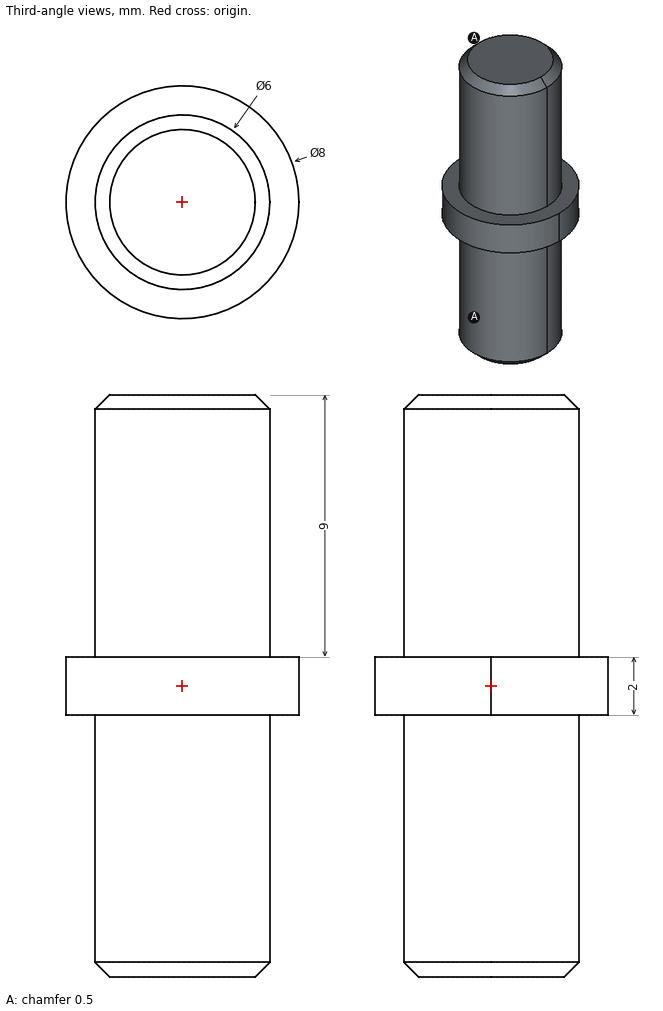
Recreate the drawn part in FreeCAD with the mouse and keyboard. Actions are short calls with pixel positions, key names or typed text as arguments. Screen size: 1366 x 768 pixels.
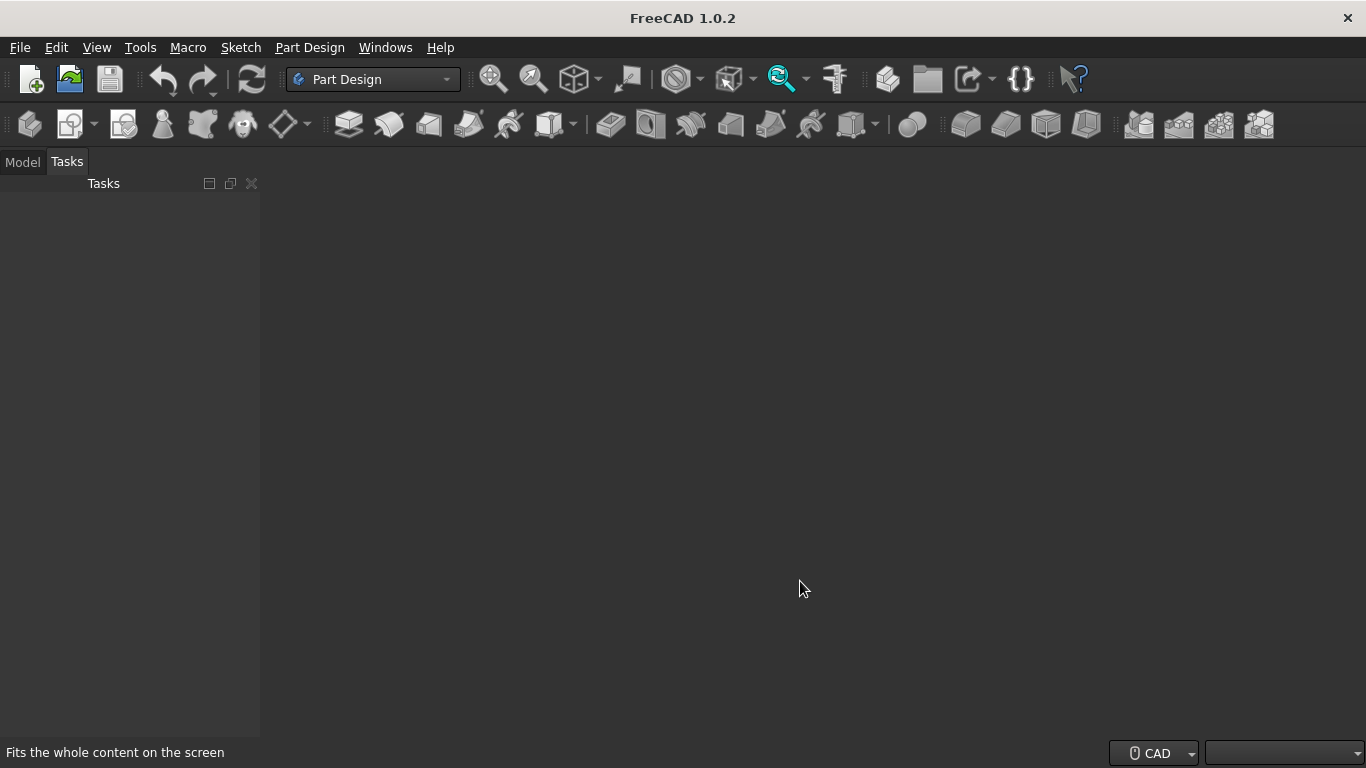
click(30, 80)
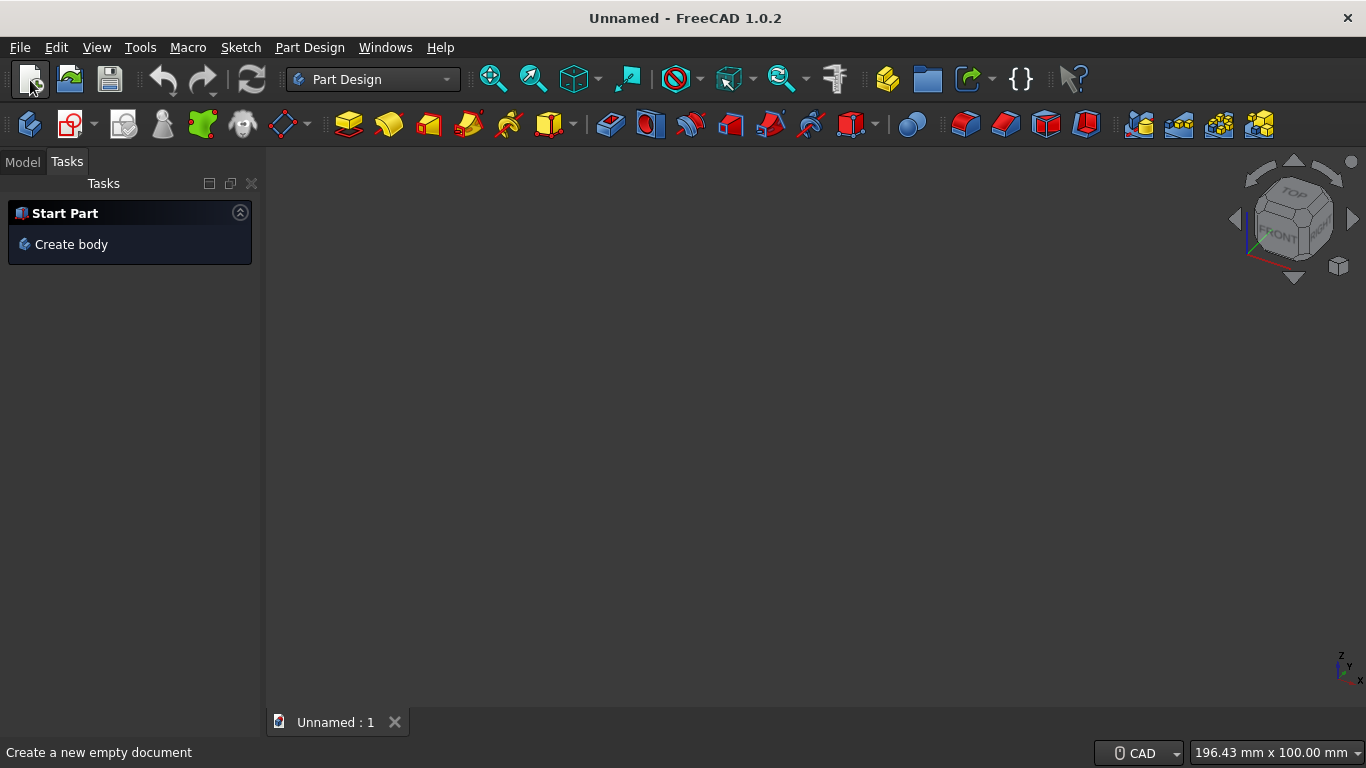
click(70, 124)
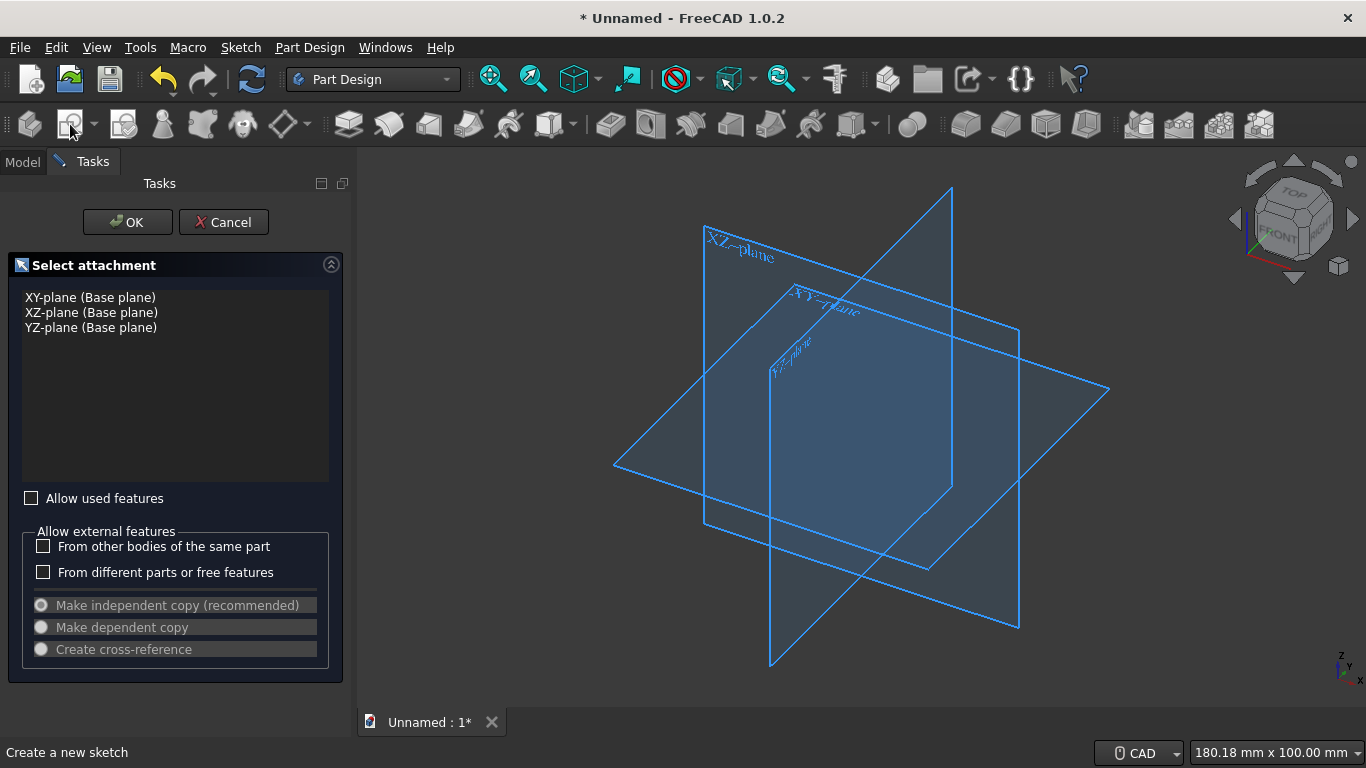
click(82, 298)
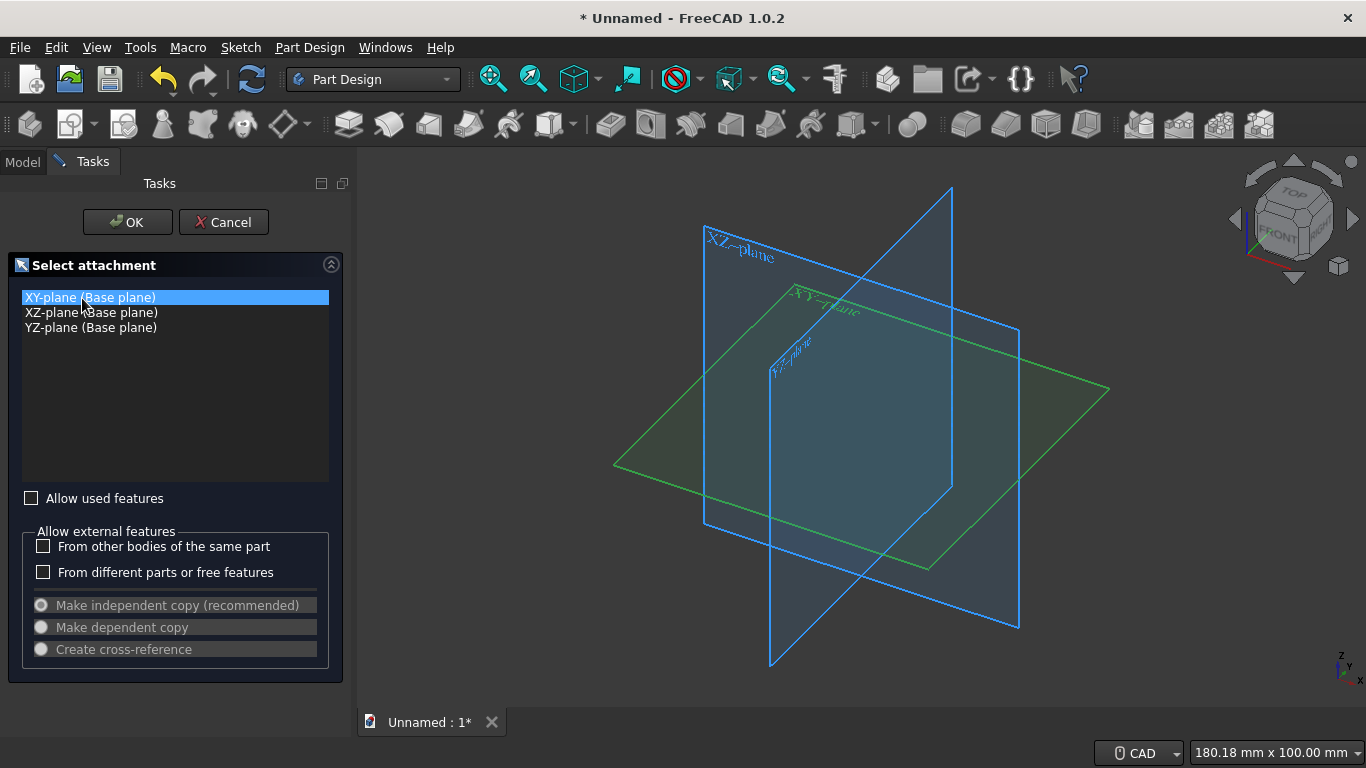
click(128, 222)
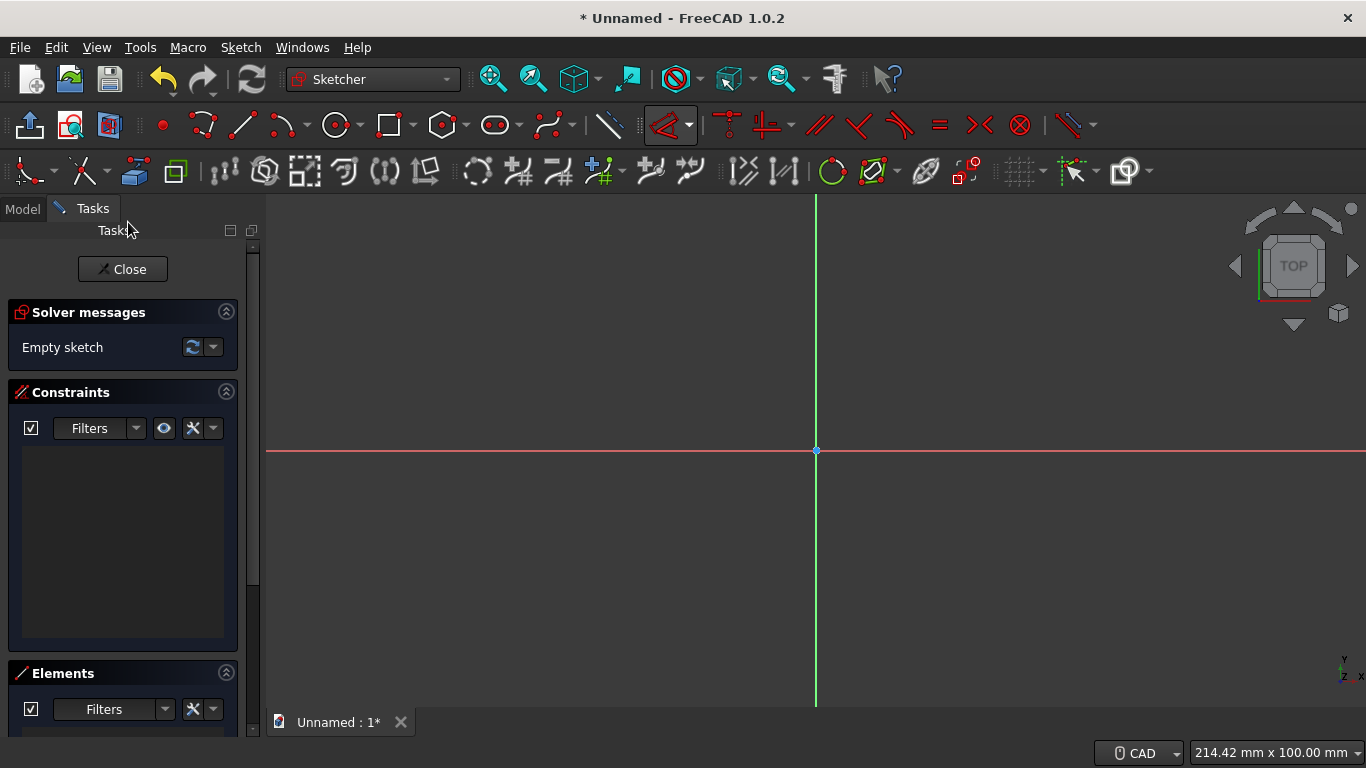
scroll(827, 450, up, 10)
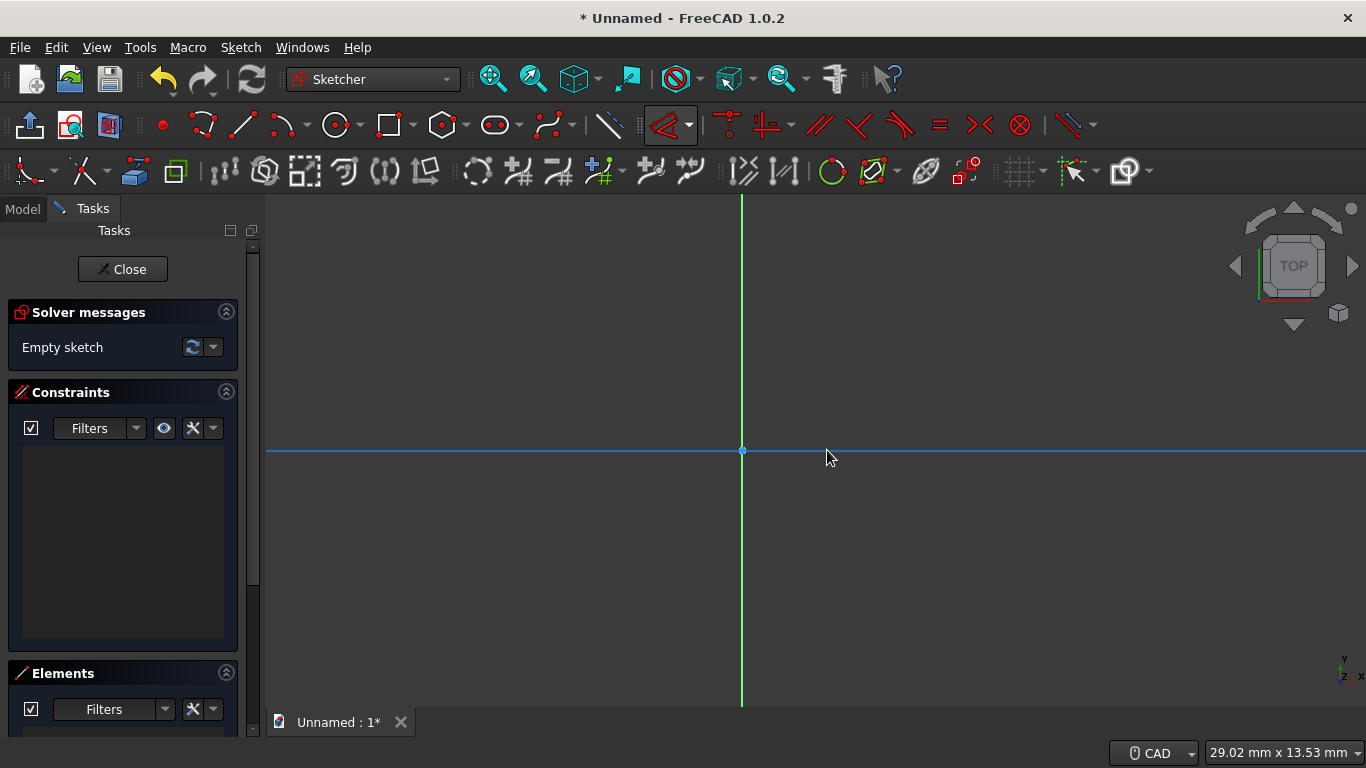
key(g)
key(c)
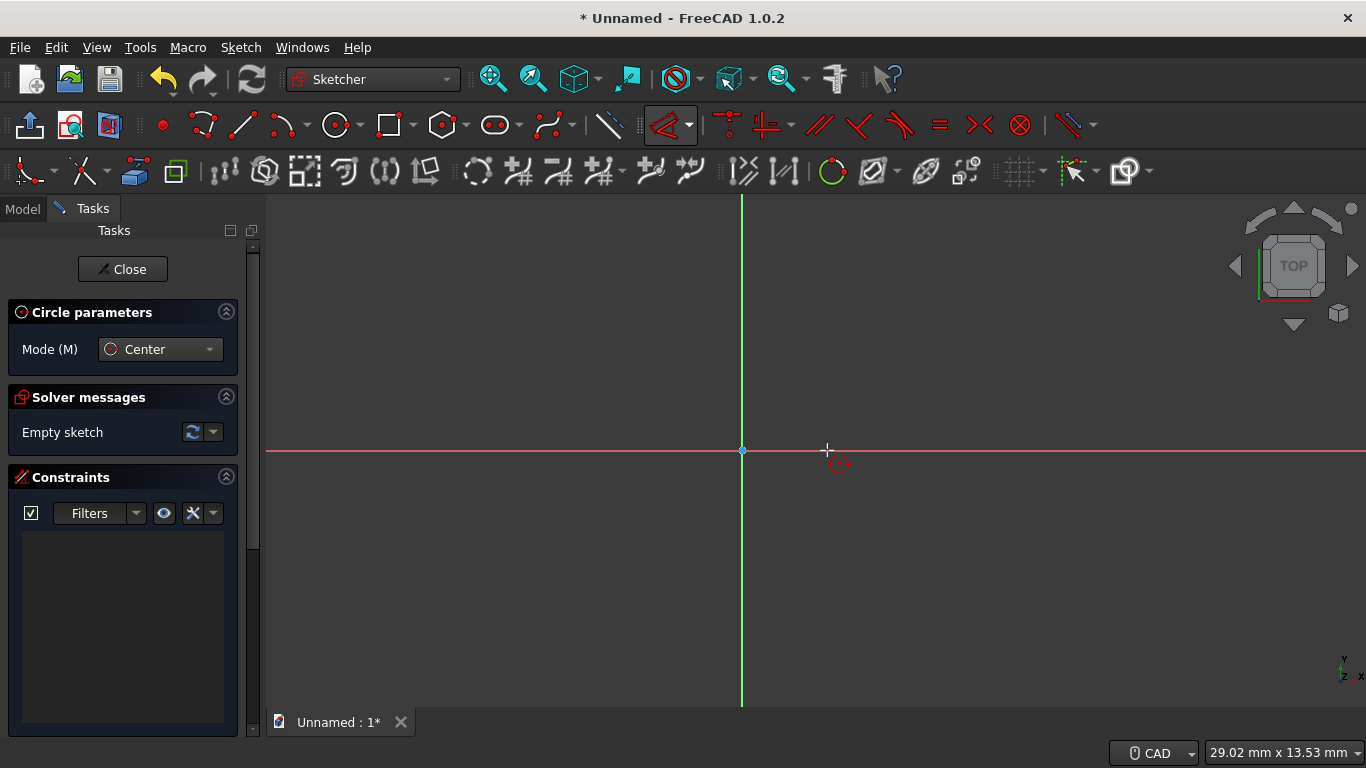
click(742, 450)
click(850, 343)
key(Escape)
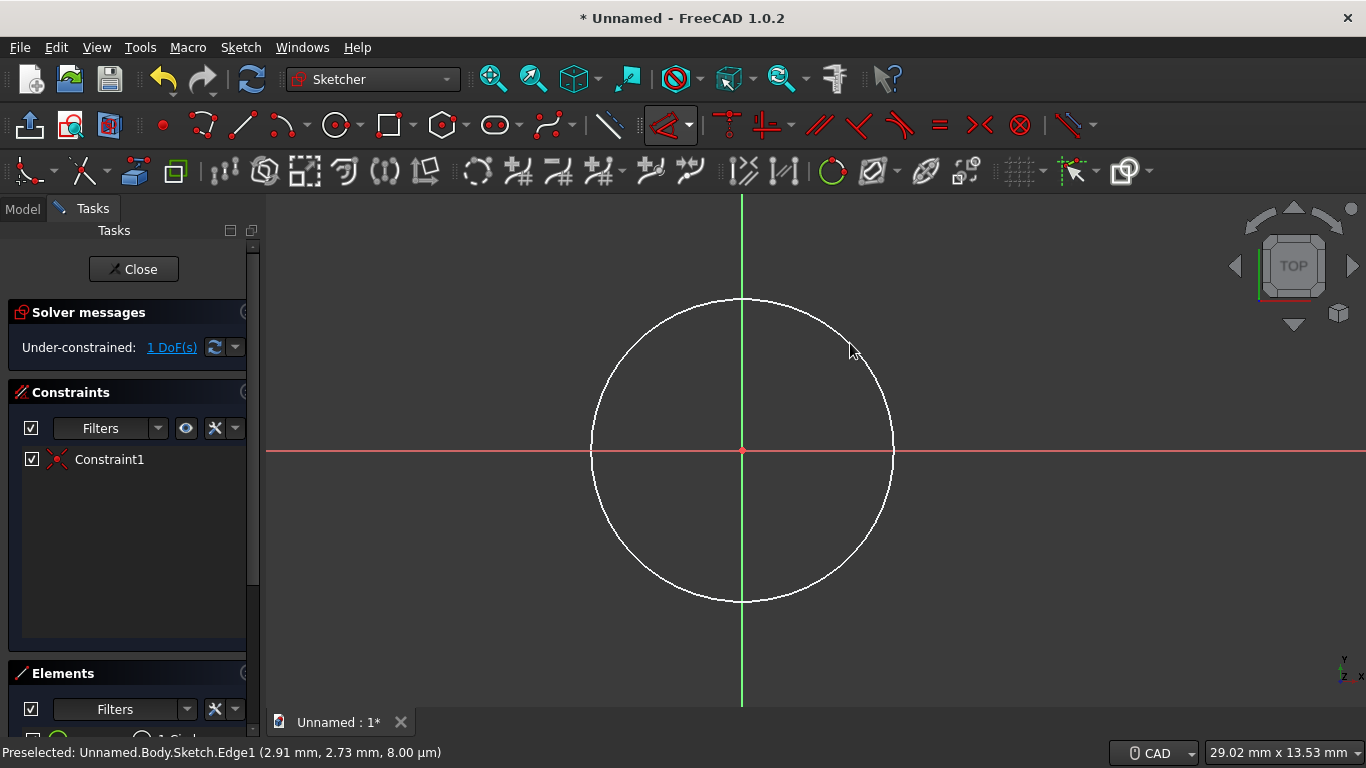
key(d)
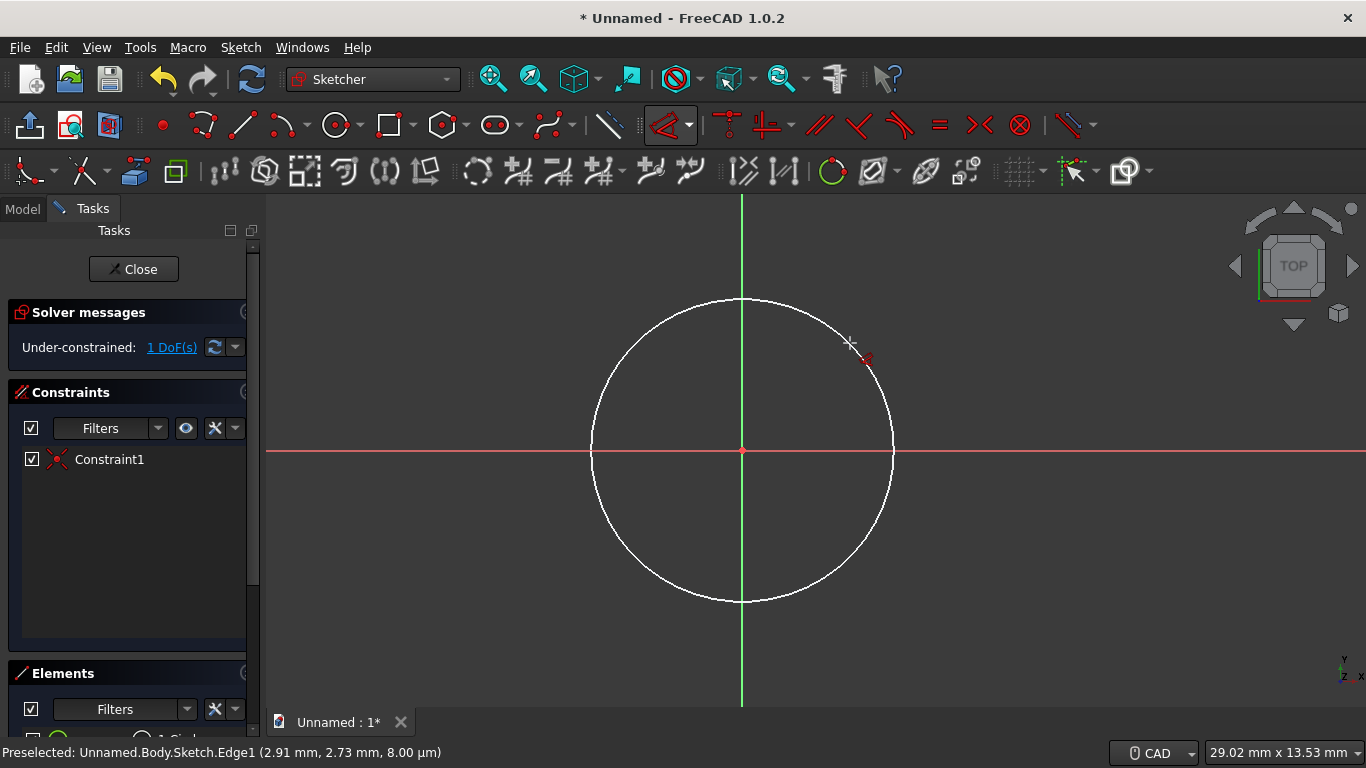
click(849, 343)
click(872, 320)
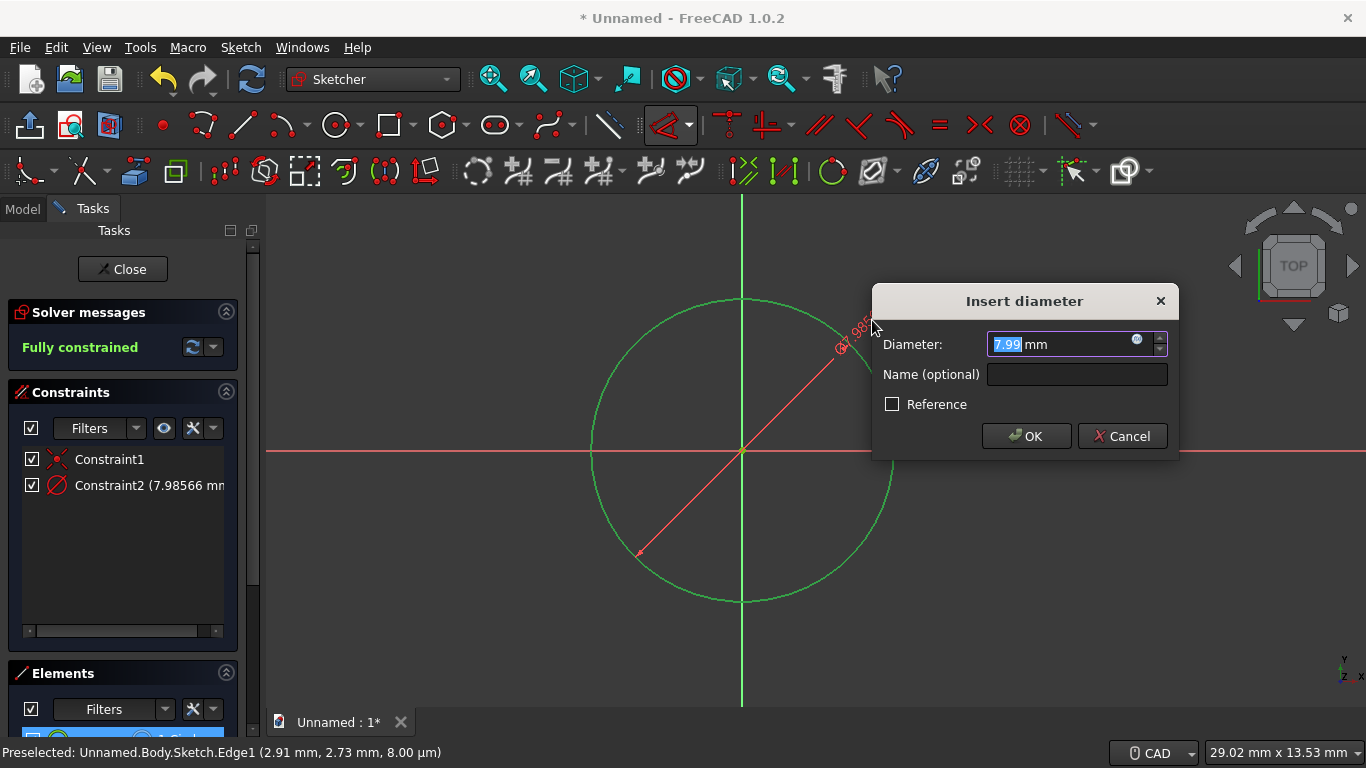
text(8)
key(Return)
key(Escape)